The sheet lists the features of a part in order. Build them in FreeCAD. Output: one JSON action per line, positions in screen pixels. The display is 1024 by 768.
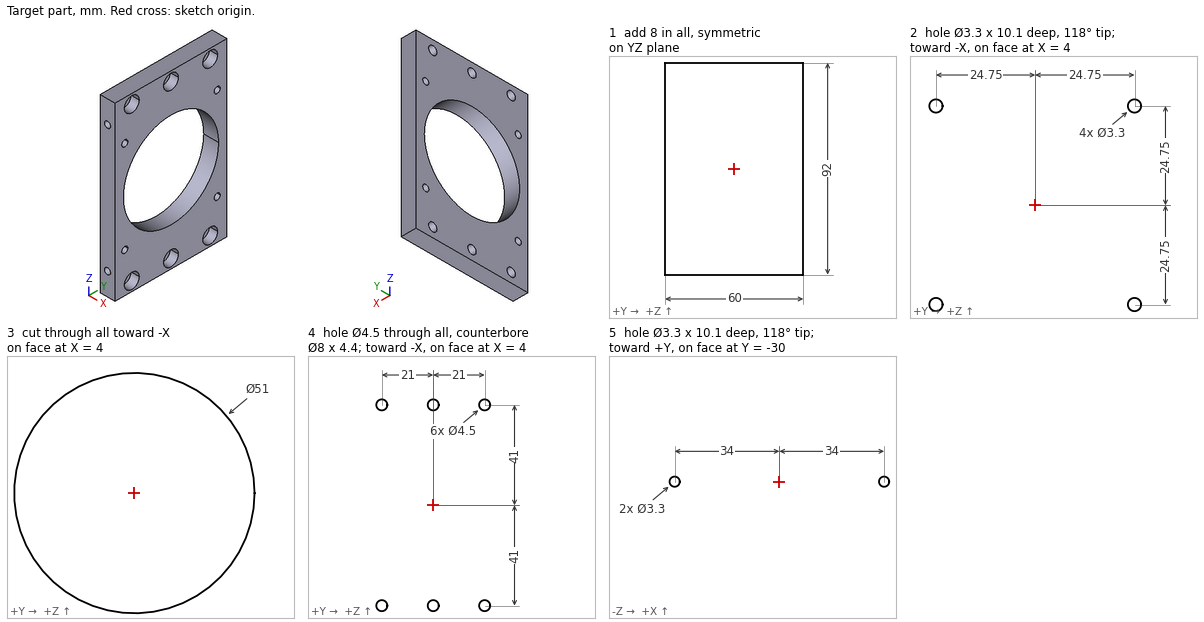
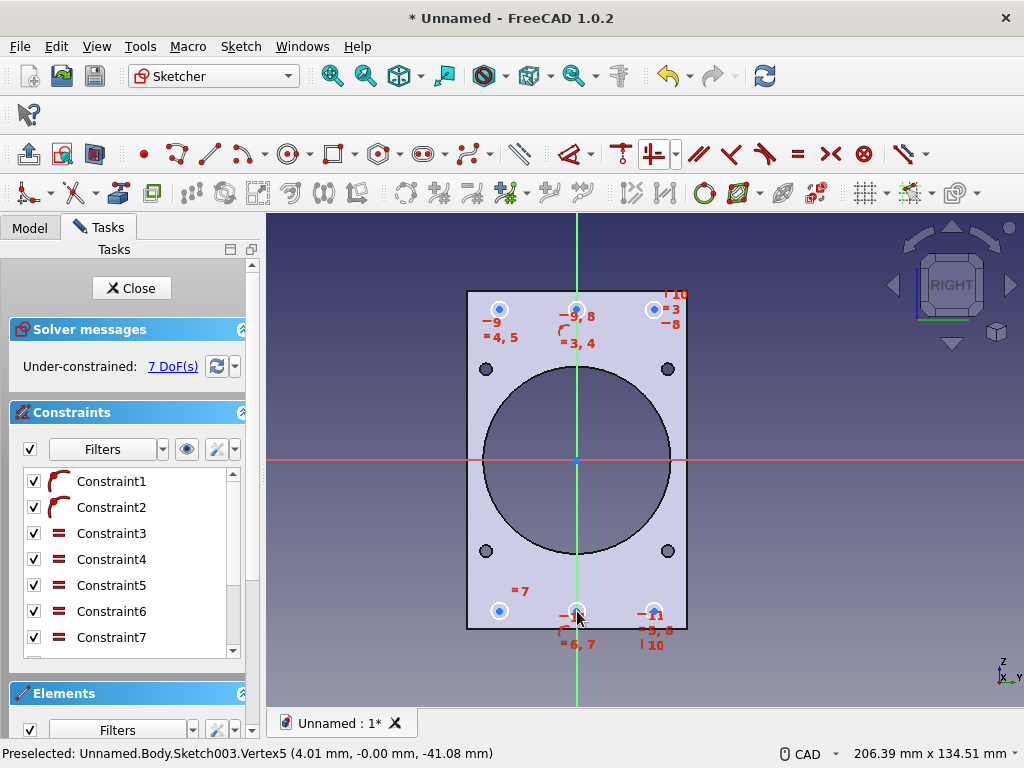
{"action": "left_click", "coordinate": [500, 310]}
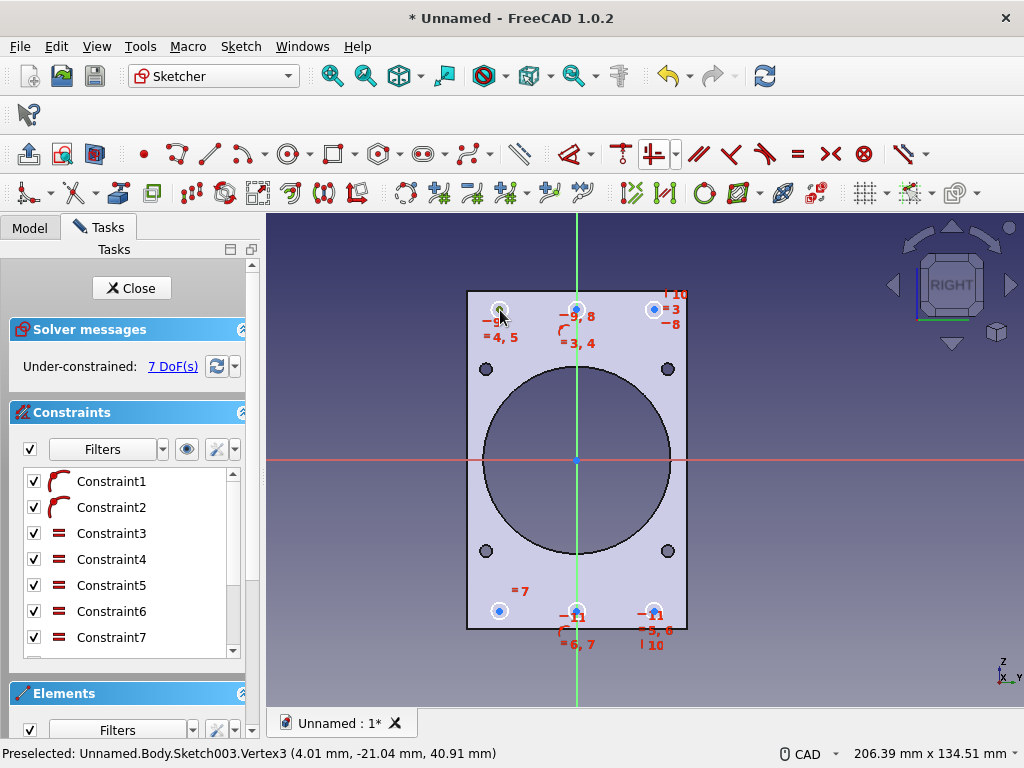
{"action": "left_click", "coordinate": [500, 611]}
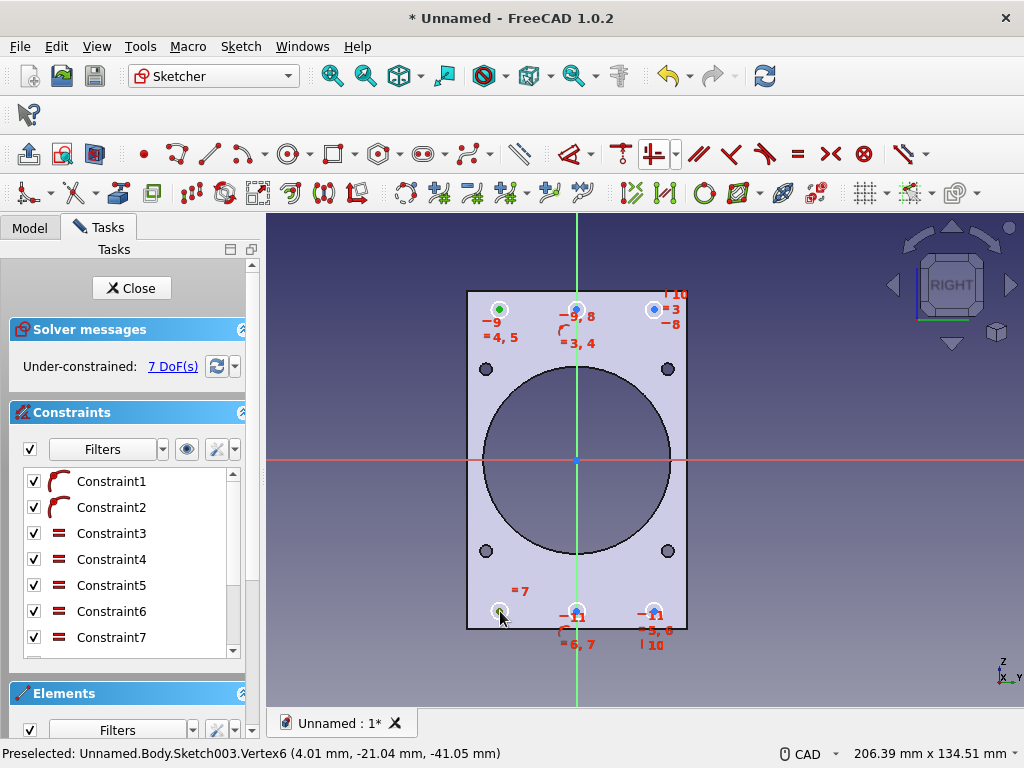
{"action": "key", "text": "v"}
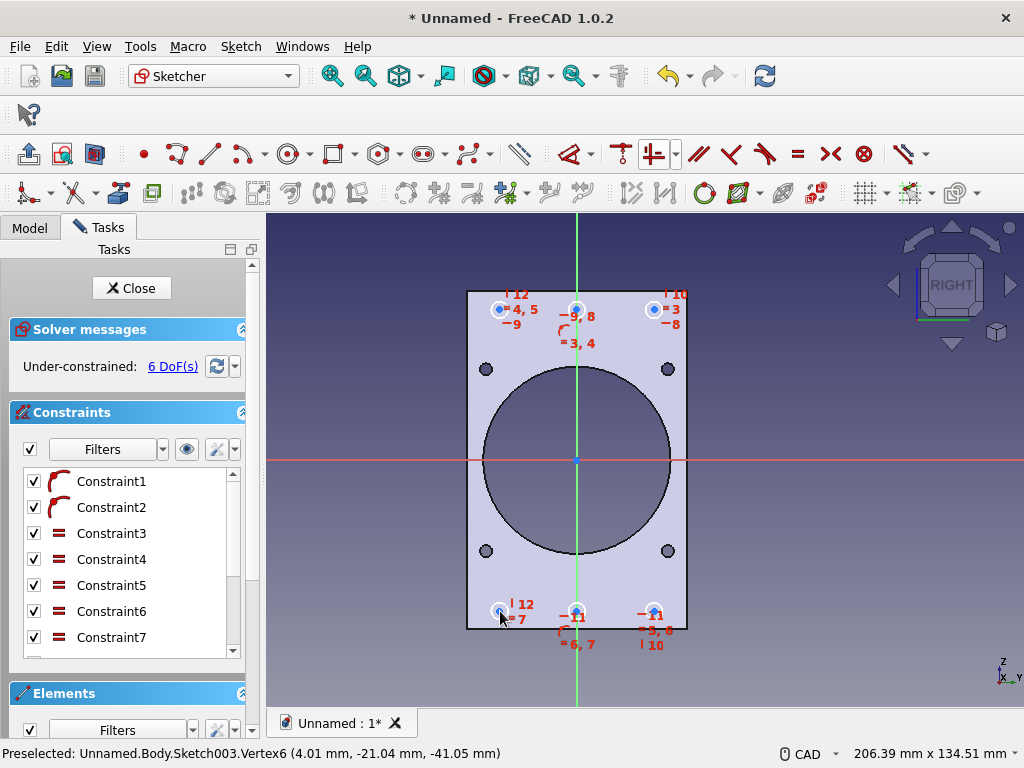
{"action": "scroll", "coordinate": [577, 611], "scroll_direction": "up", "scroll_amount": 4}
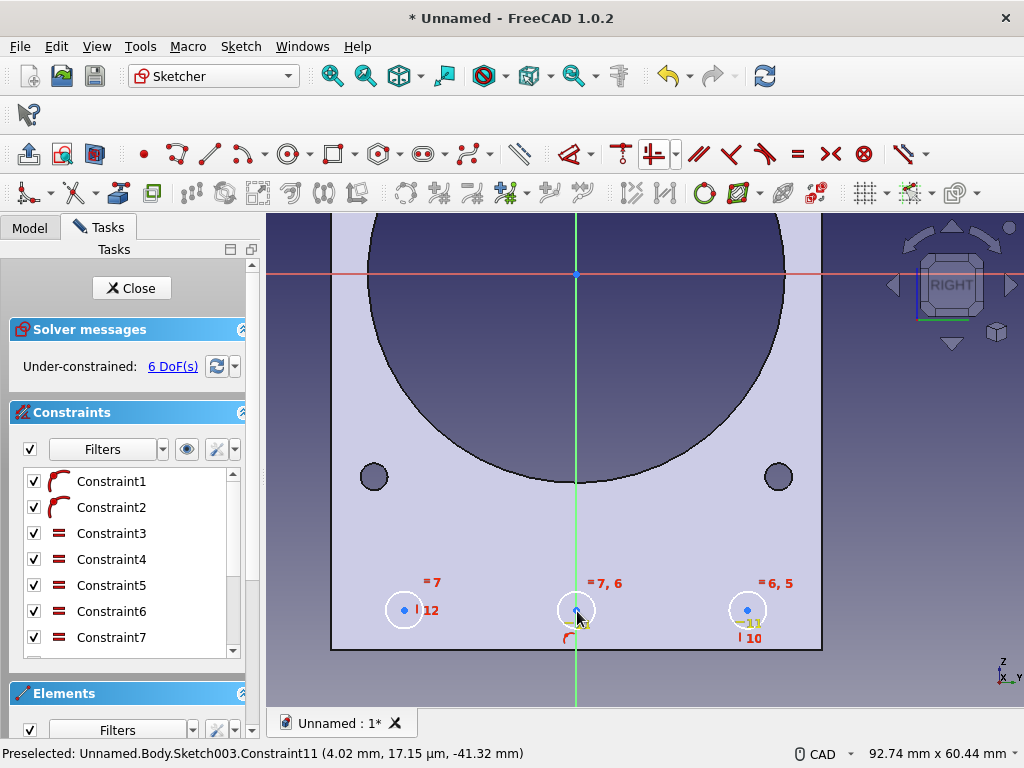
{"action": "left_click", "coordinate": [576, 610]}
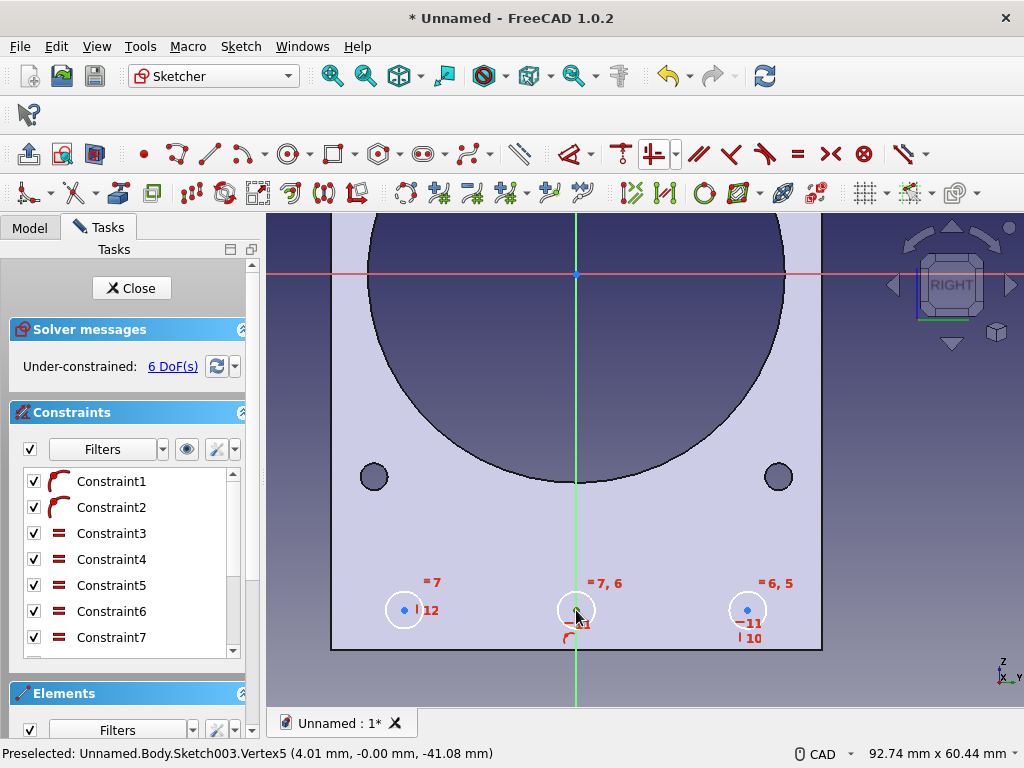
{"action": "left_click", "coordinate": [404, 610]}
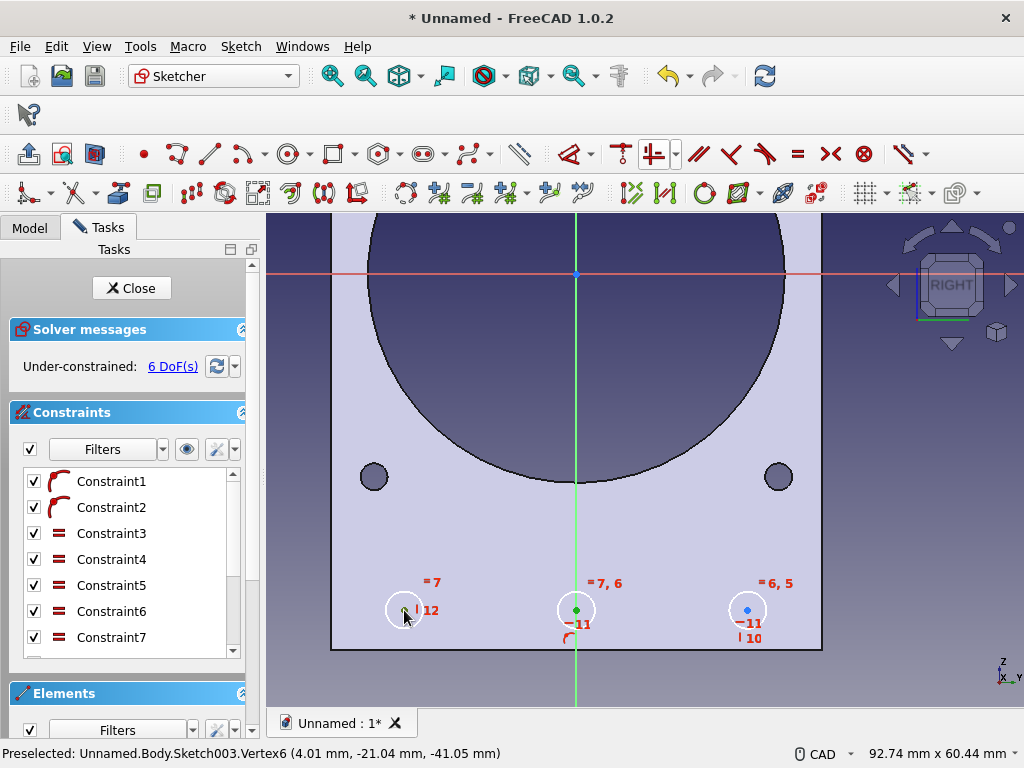
{"action": "left_click", "coordinate": [676, 154]}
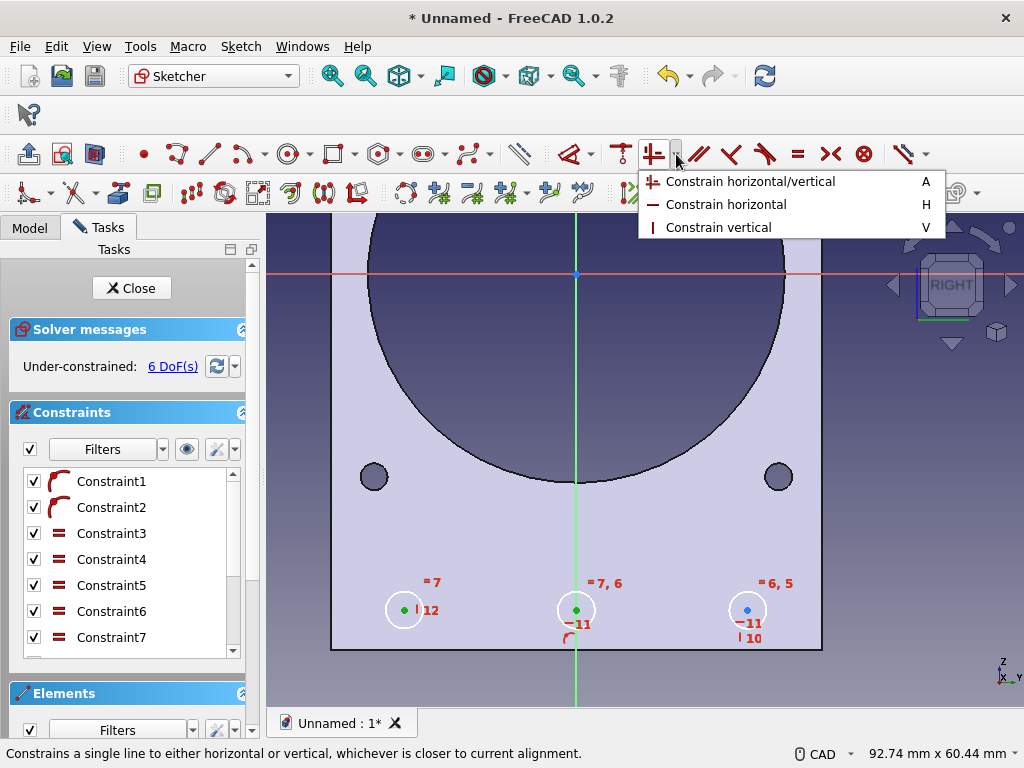
{"action": "left_click", "coordinate": [792, 204]}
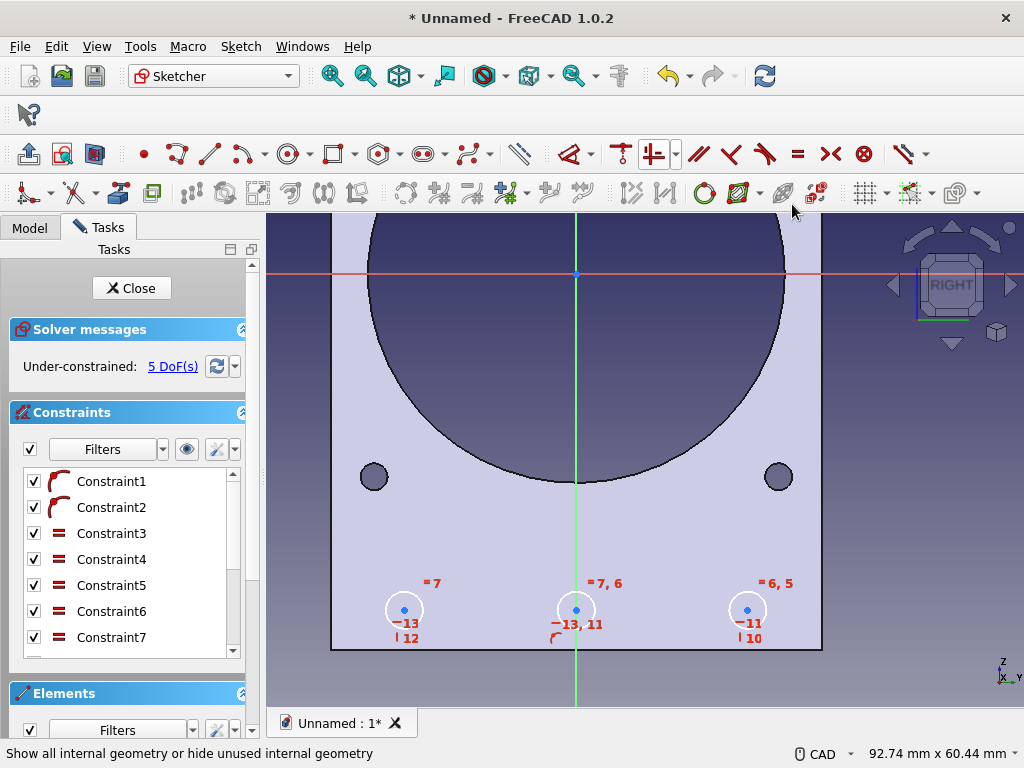
{"action": "left_click", "coordinate": [568, 154]}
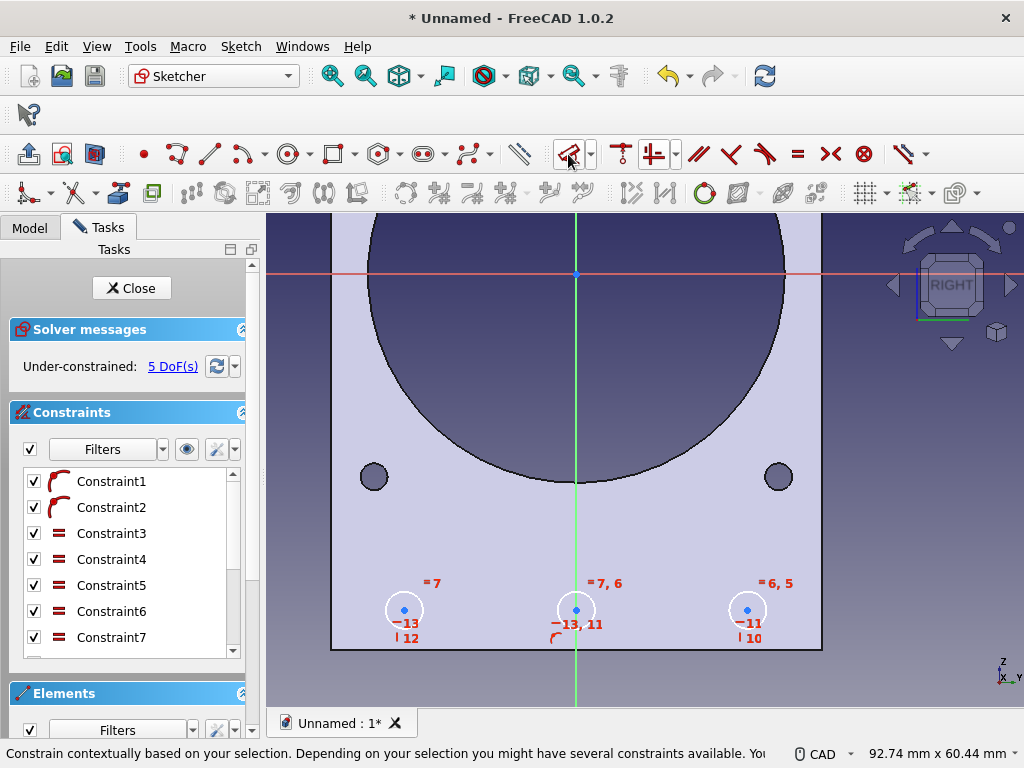
{"action": "scroll", "coordinate": [577, 611], "scroll_direction": "down", "scroll_amount": 4}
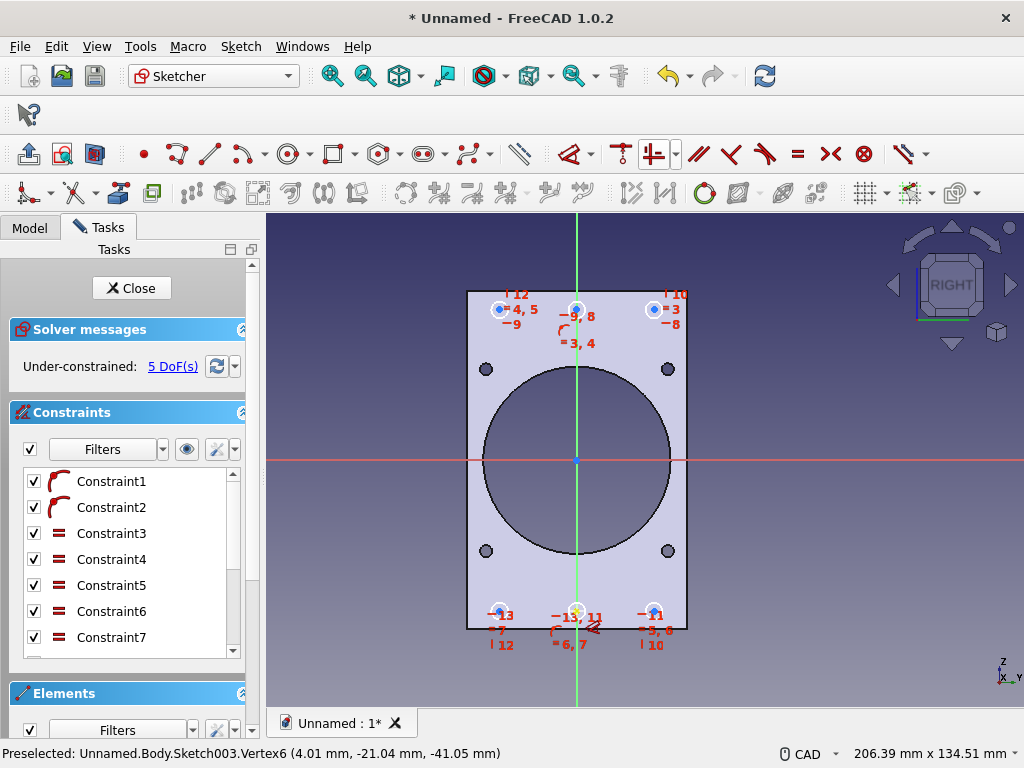
{"action": "scroll", "coordinate": [660, 304], "scroll_direction": "up", "scroll_amount": 5}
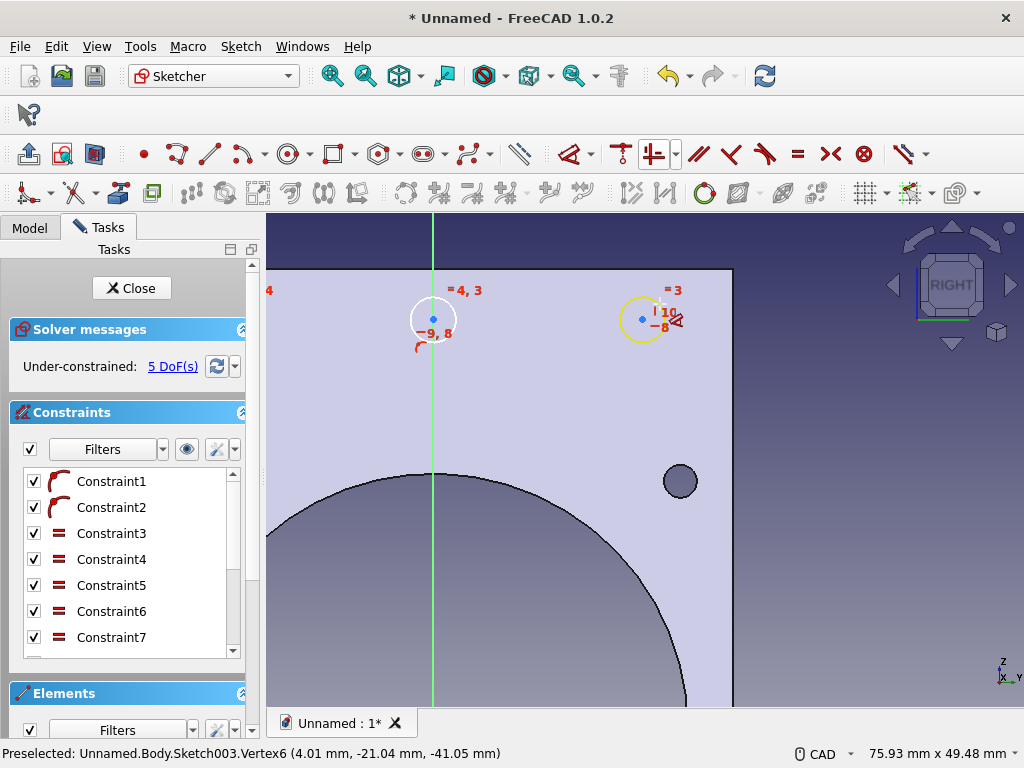
{"action": "left_click", "coordinate": [659, 304]}
{"action": "left_click", "coordinate": [682, 282]}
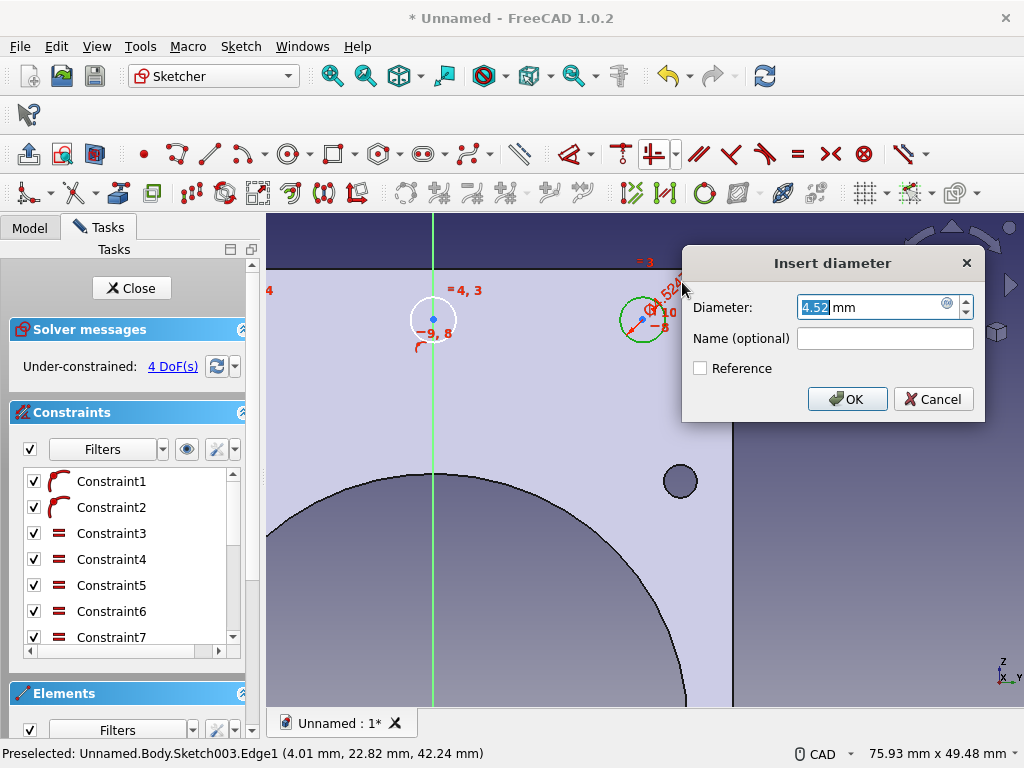
{"action": "type", "text": "4.5"}
{"action": "key", "text": "Return"}